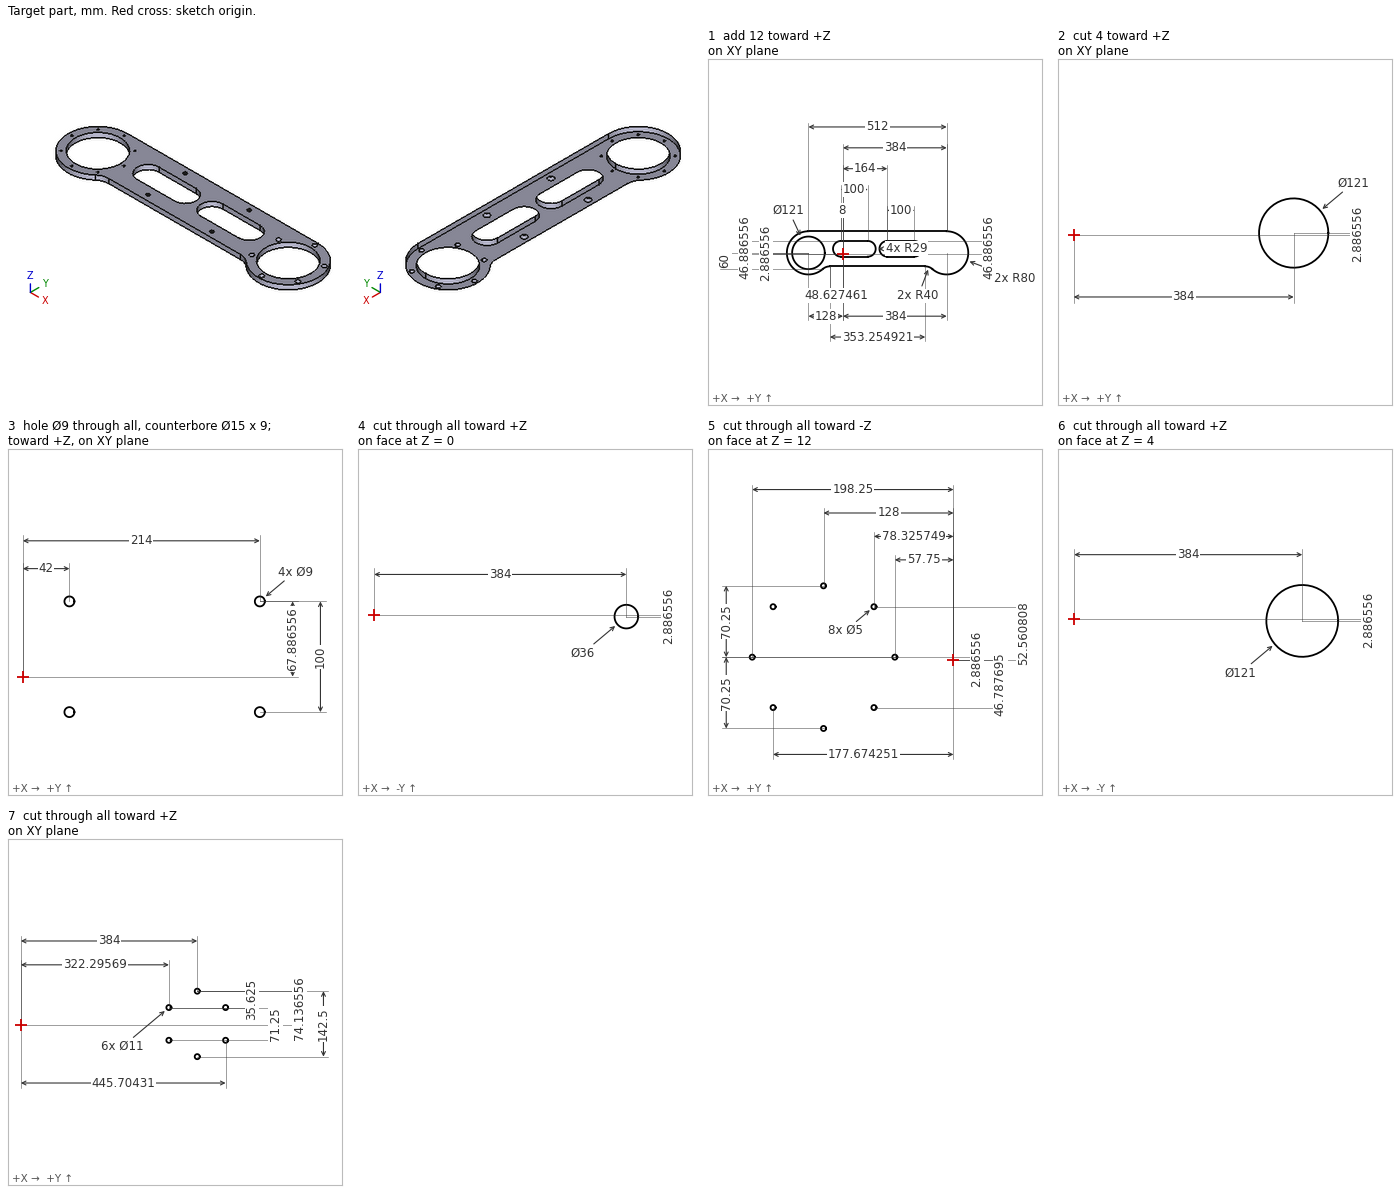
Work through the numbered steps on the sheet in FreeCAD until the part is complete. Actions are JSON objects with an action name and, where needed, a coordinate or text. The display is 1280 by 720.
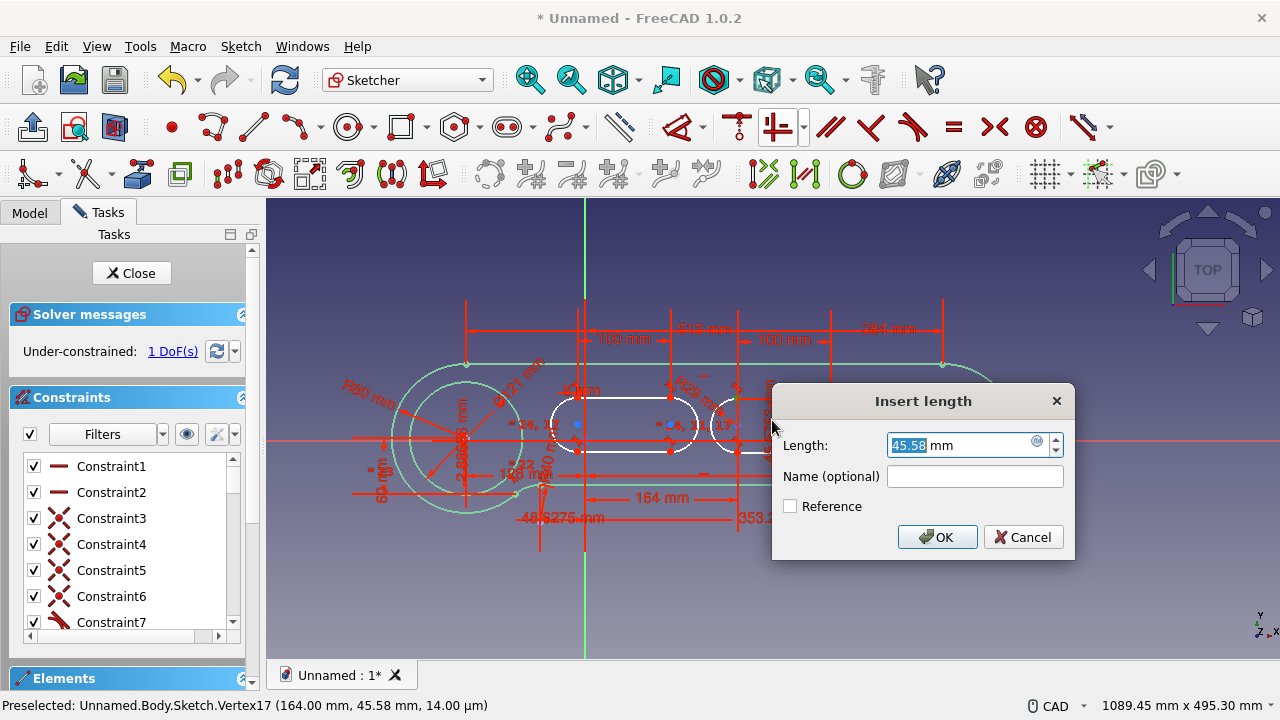
{"action": "type", "text": "46.886556"}
{"action": "key", "text": "Return"}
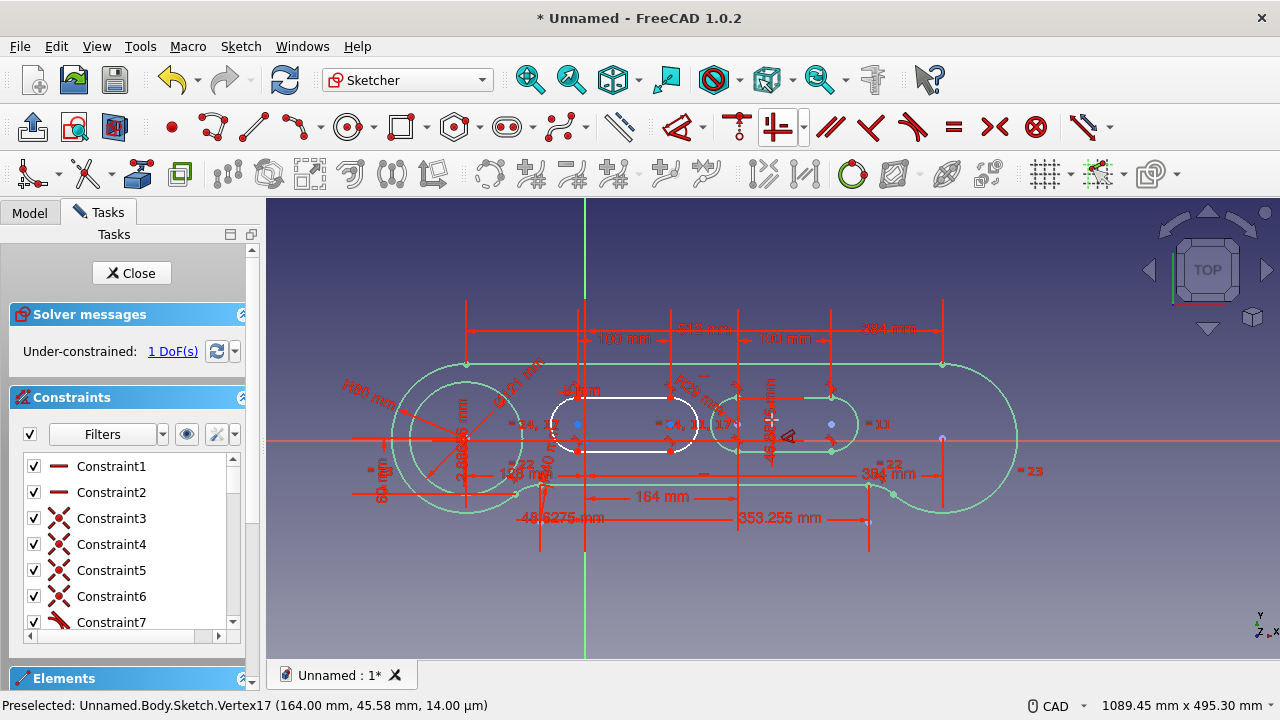
{"action": "left_click", "coordinate": [578, 398]}
{"action": "left_click", "coordinate": [619, 420]}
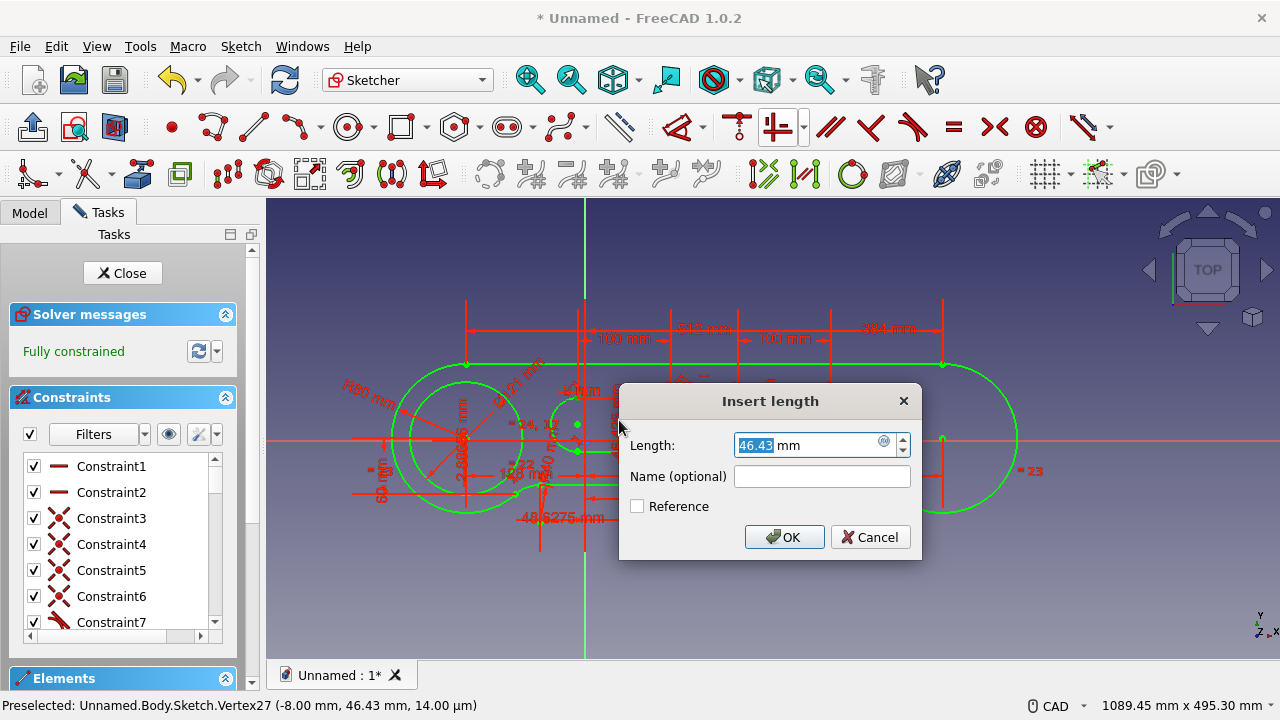
{"action": "type", "text": "46.886556"}
{"action": "key", "text": "Return"}
{"action": "key", "text": "Escape"}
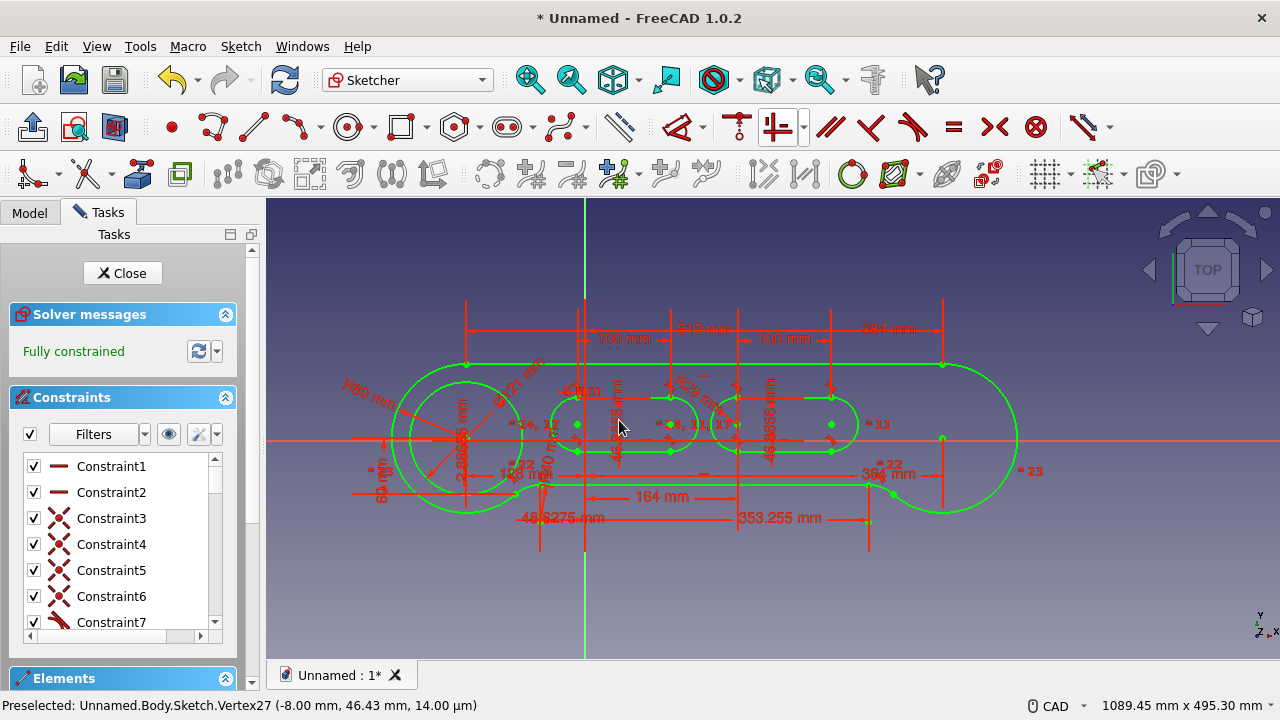
{"action": "left_click", "coordinate": [123, 273]}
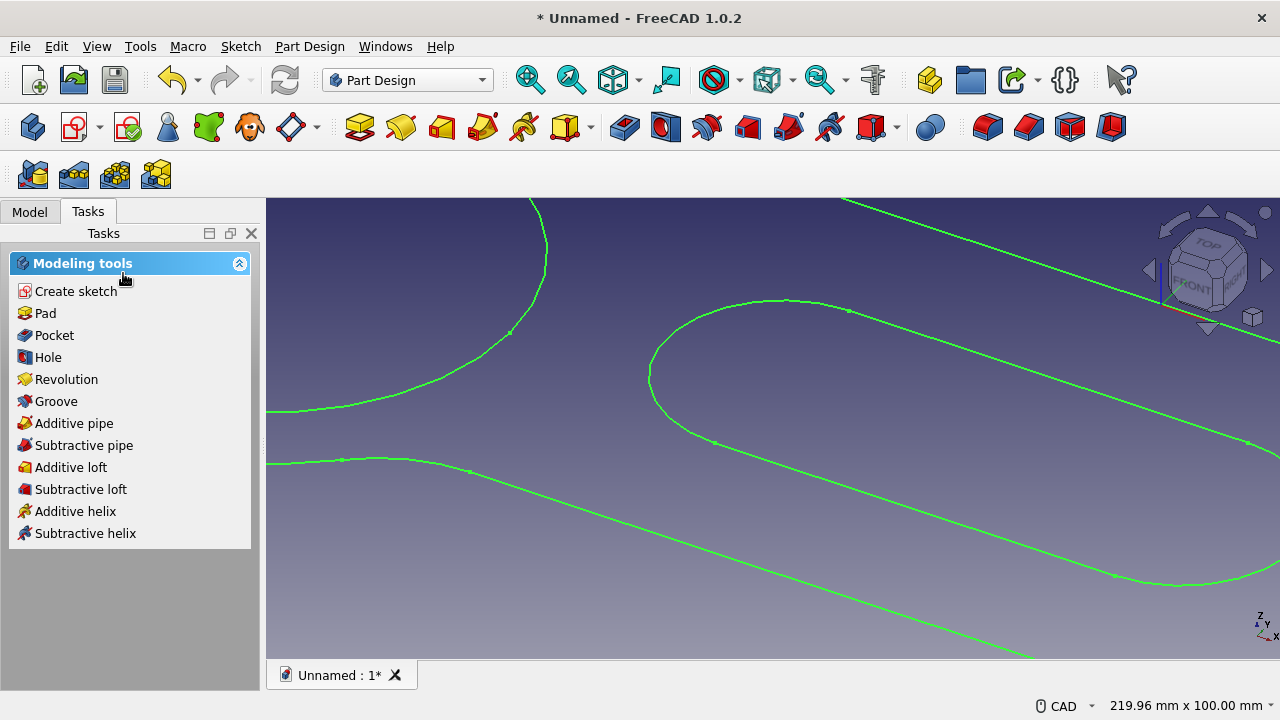
{"action": "left_click", "coordinate": [360, 128]}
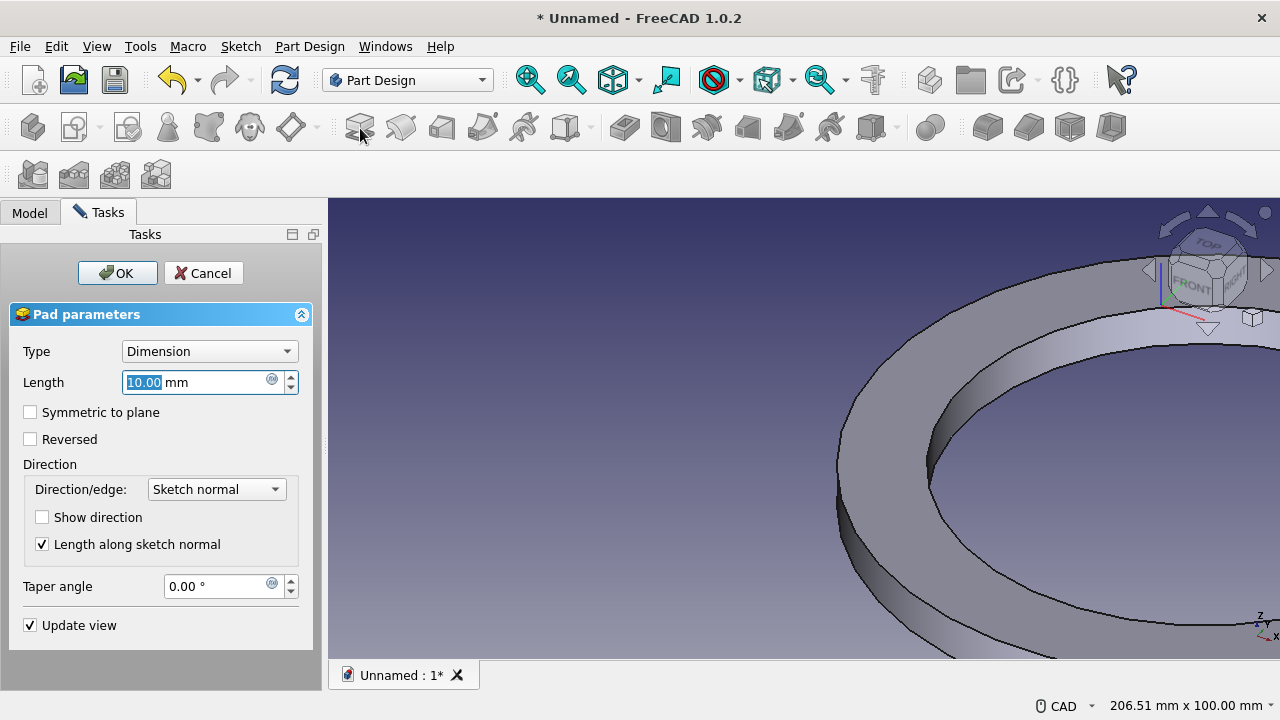
{"action": "type", "text": "12"}
{"action": "key", "text": "Tab"}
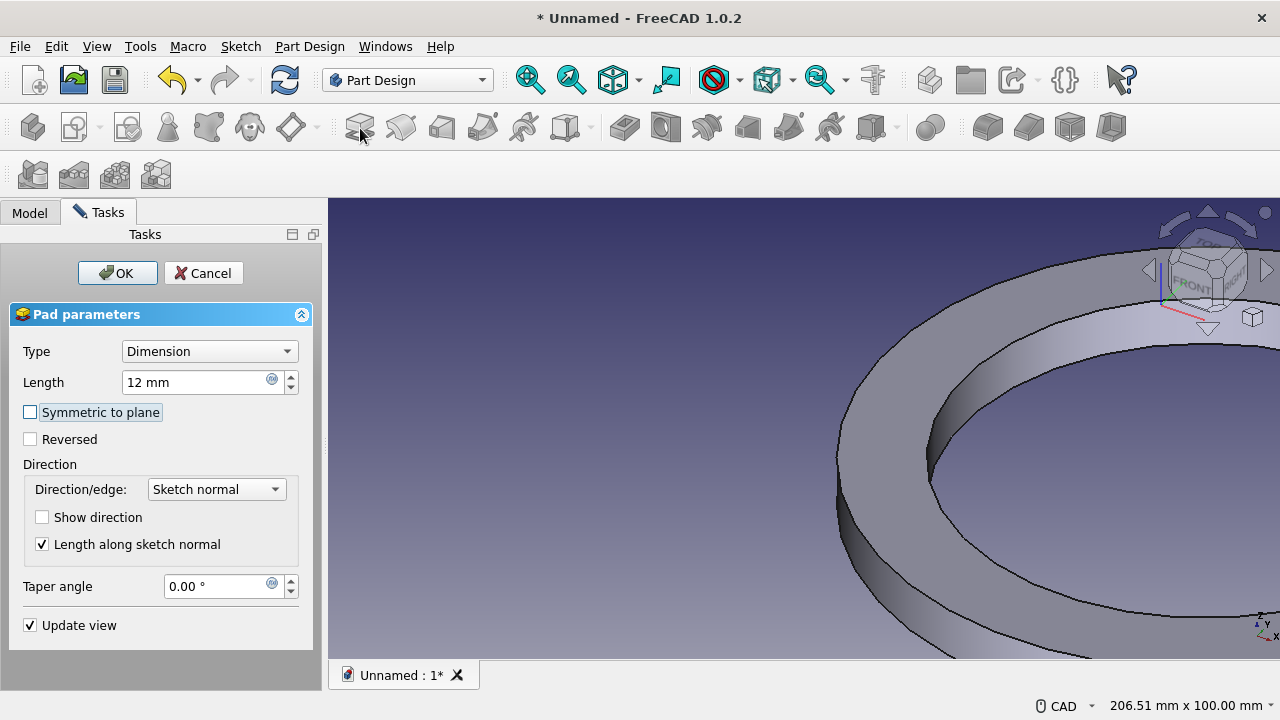
{"action": "left_click", "coordinate": [118, 273]}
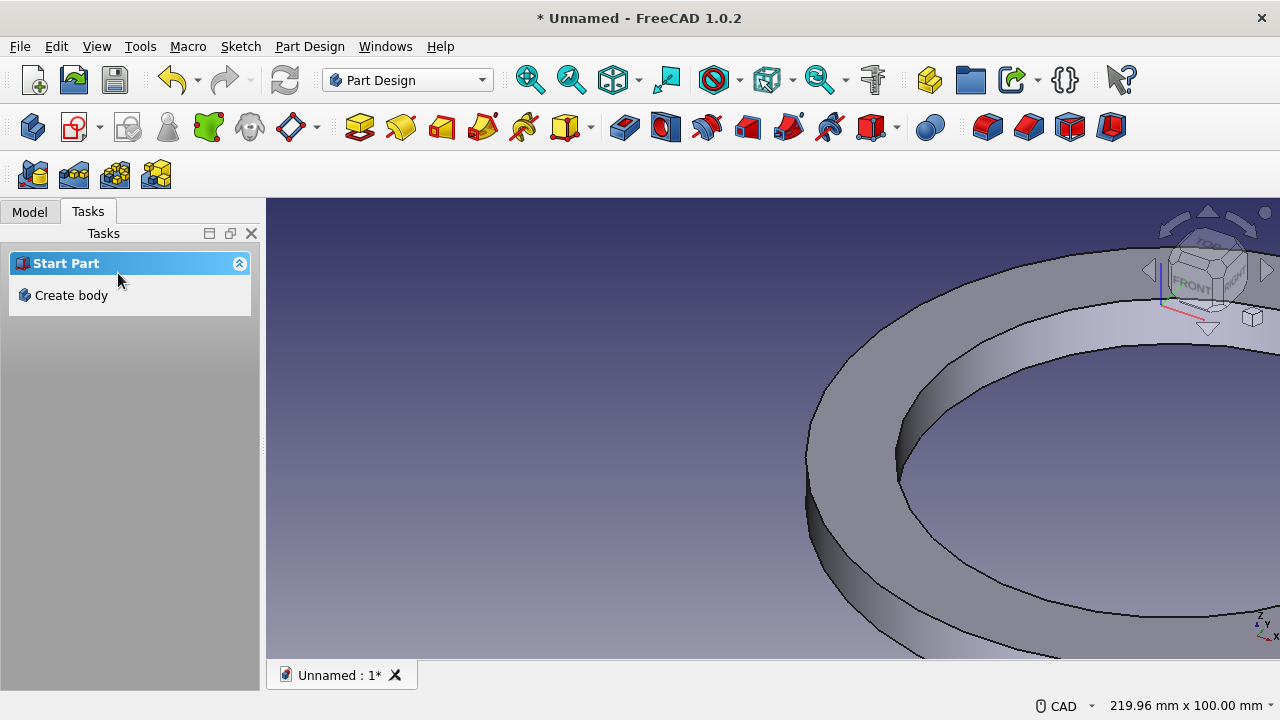
{"action": "left_click", "coordinate": [531, 80]}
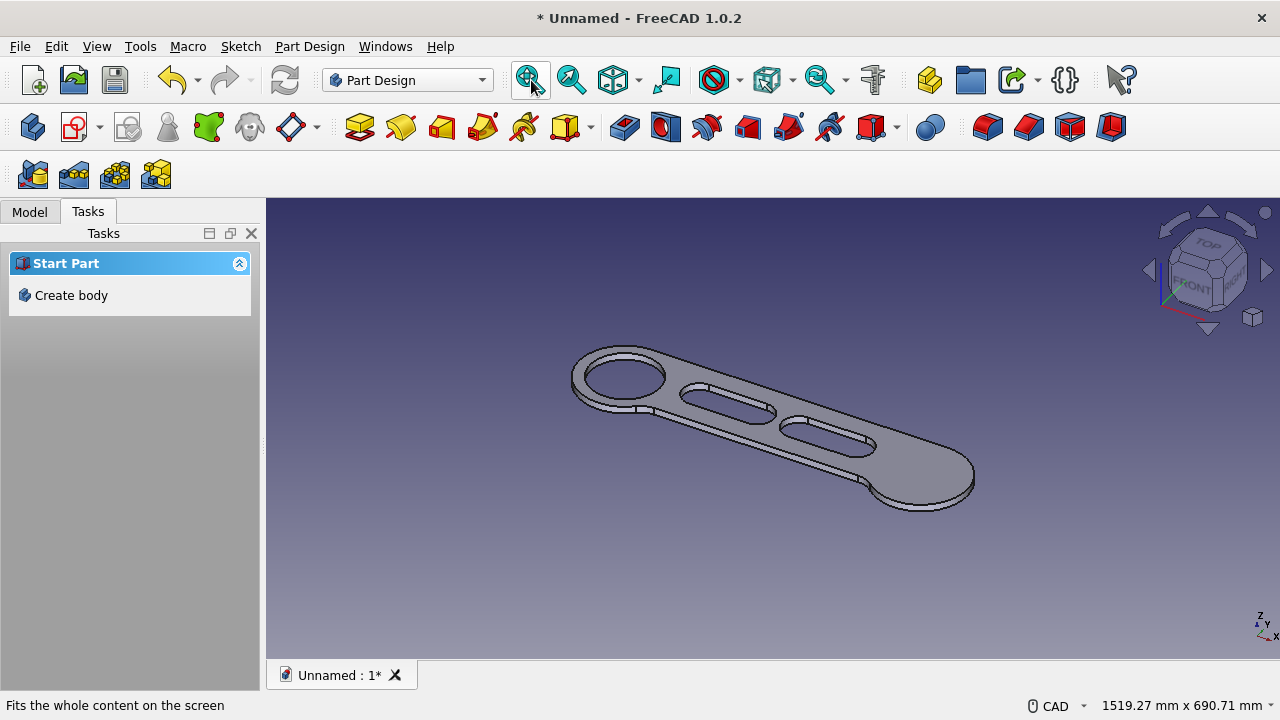
{"action": "left_click", "coordinate": [74, 128]}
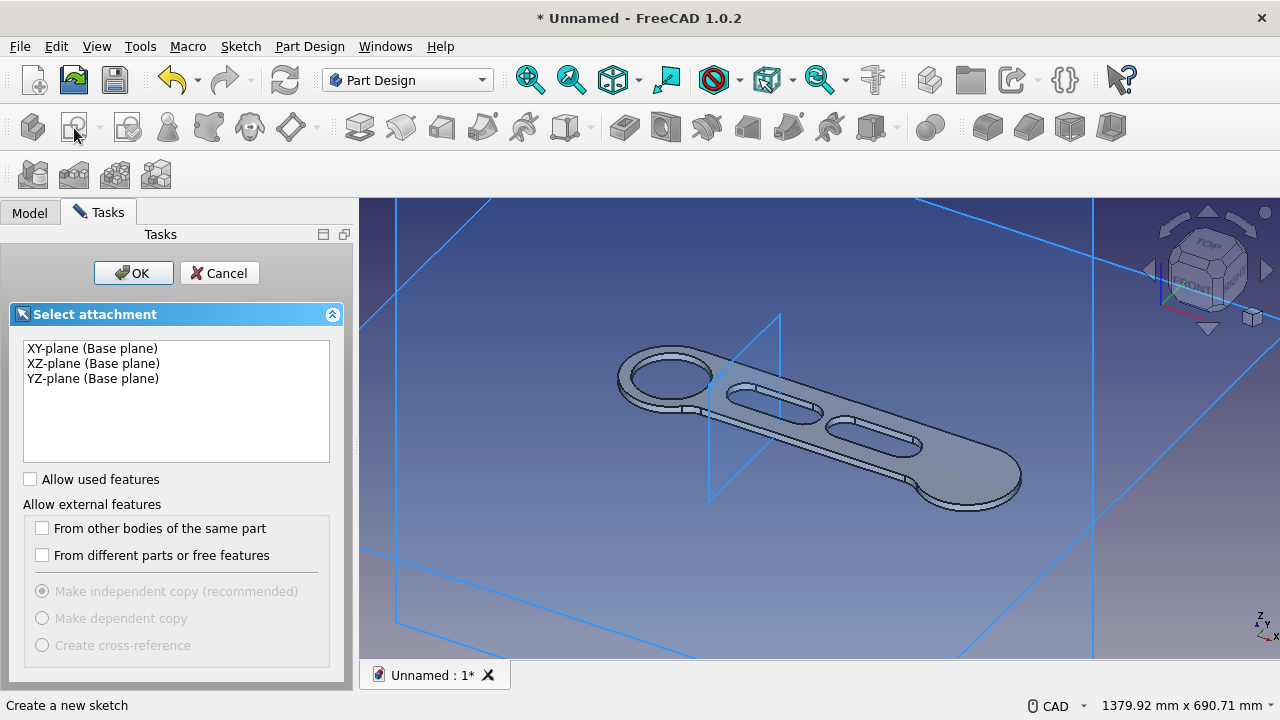
{"action": "left_click", "coordinate": [84, 348]}